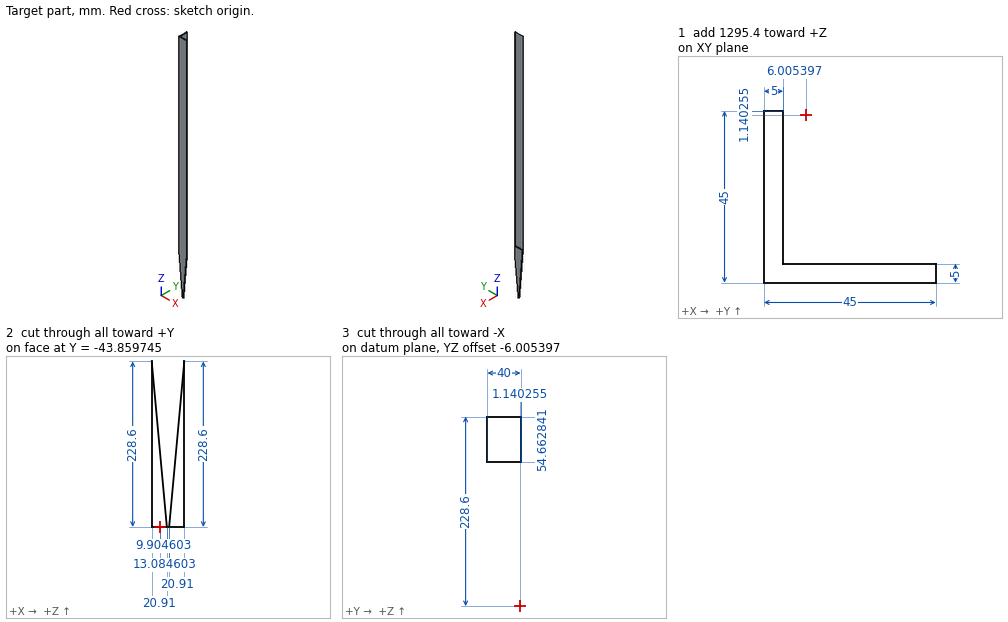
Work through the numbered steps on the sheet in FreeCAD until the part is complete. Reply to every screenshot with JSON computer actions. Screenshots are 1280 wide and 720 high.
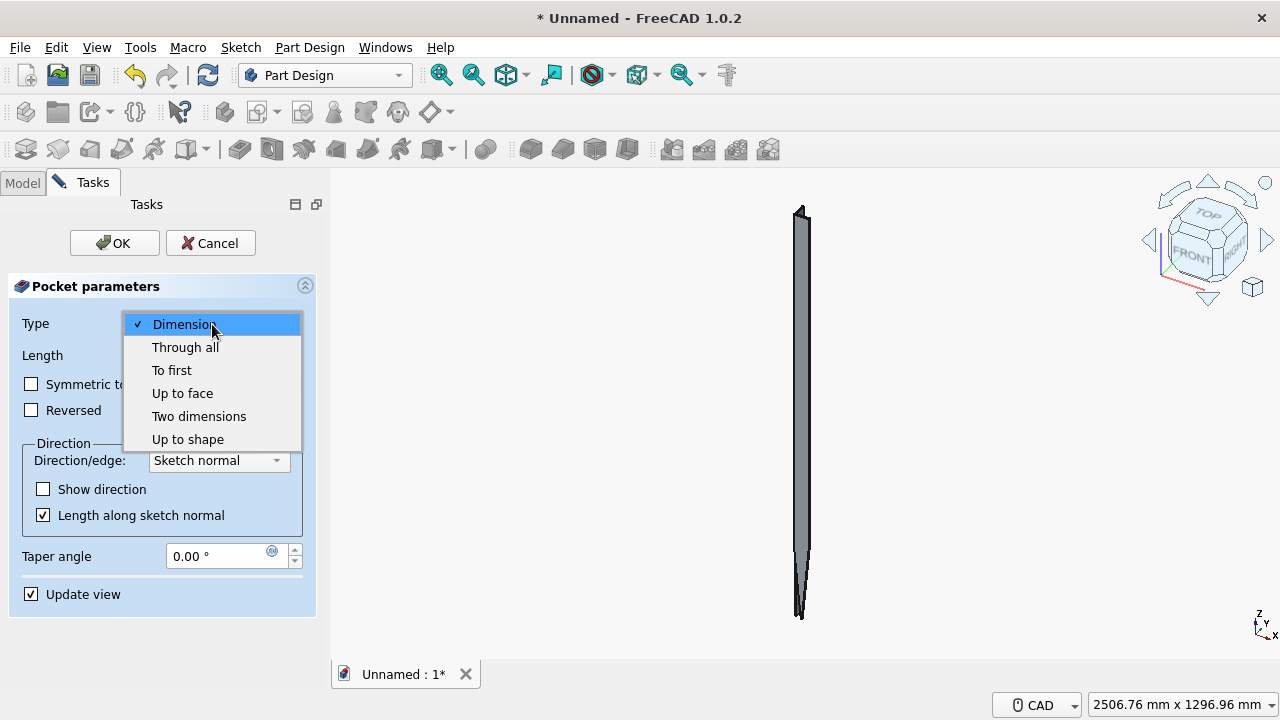
{"action": "left_click", "coordinate": [212, 348]}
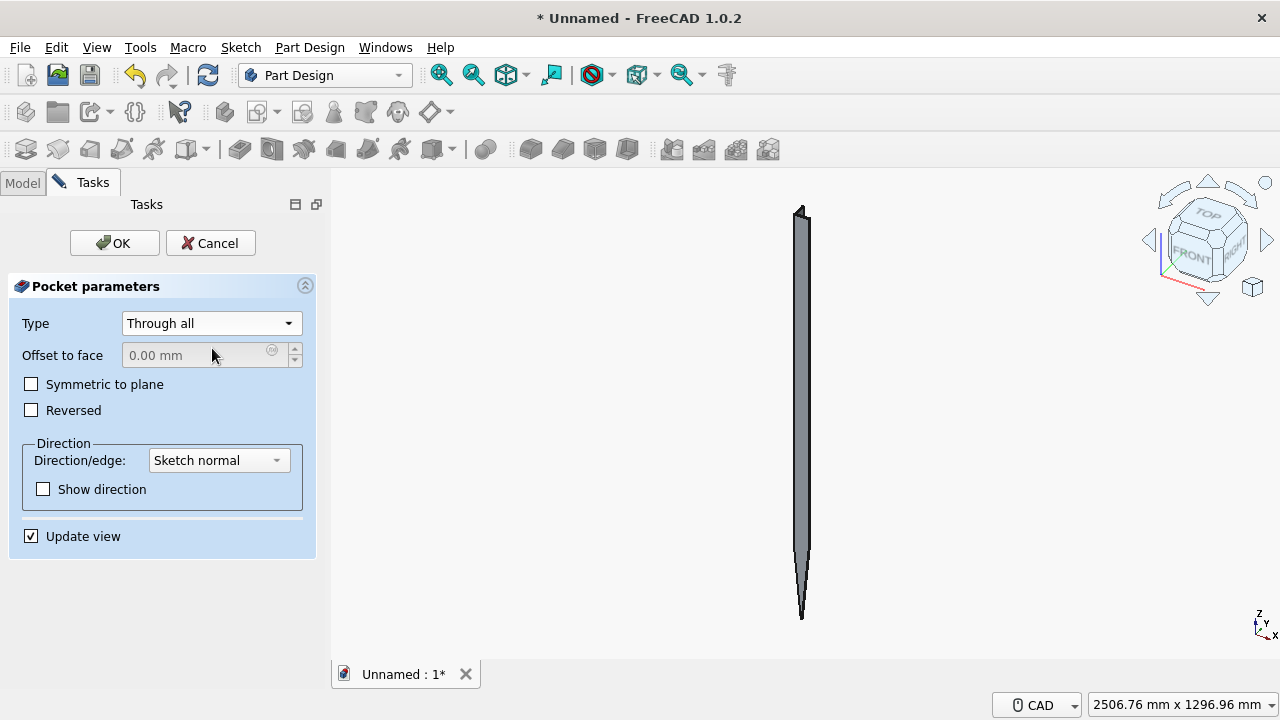
{"action": "left_click", "coordinate": [115, 243]}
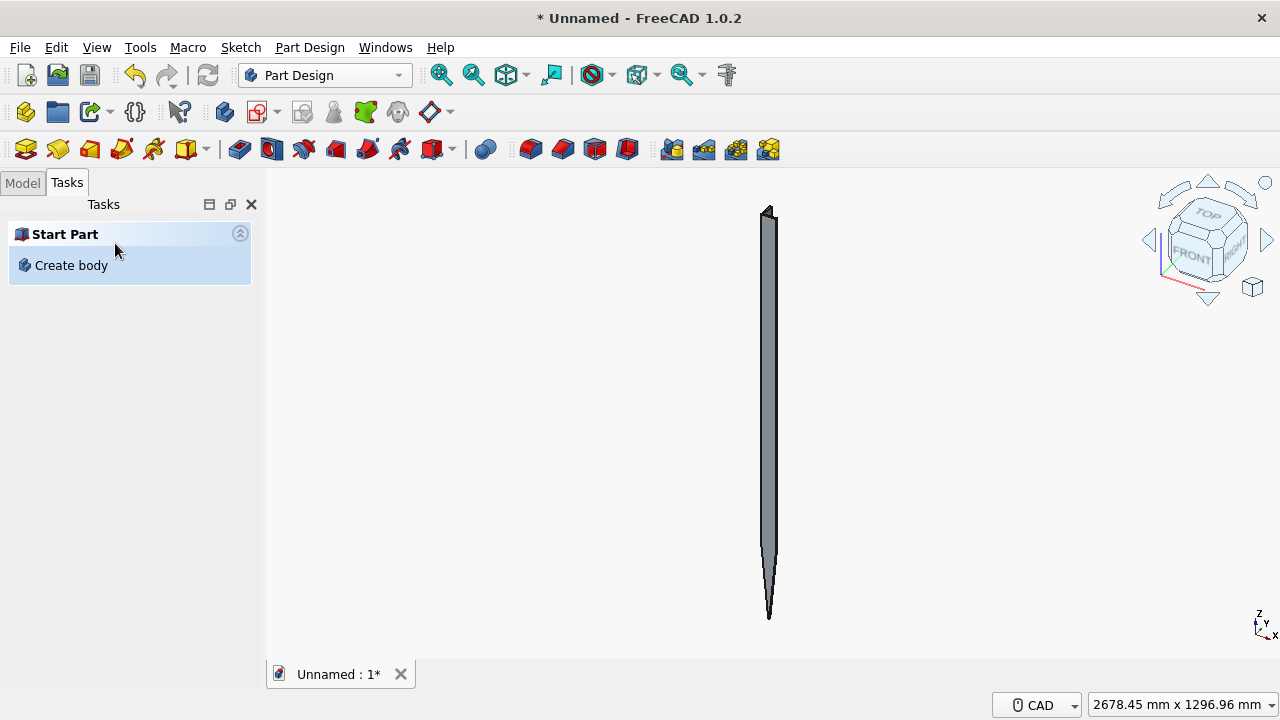
{"action": "key", "text": "0"}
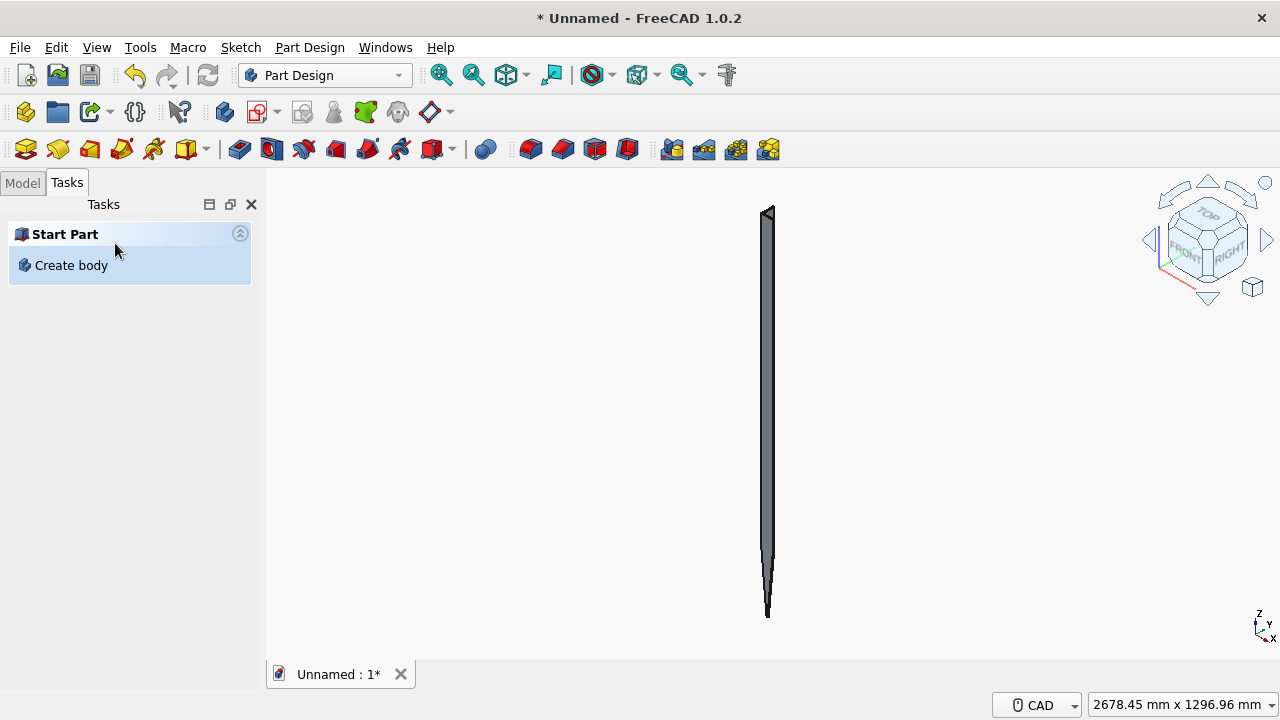
{"action": "key", "text": "3"}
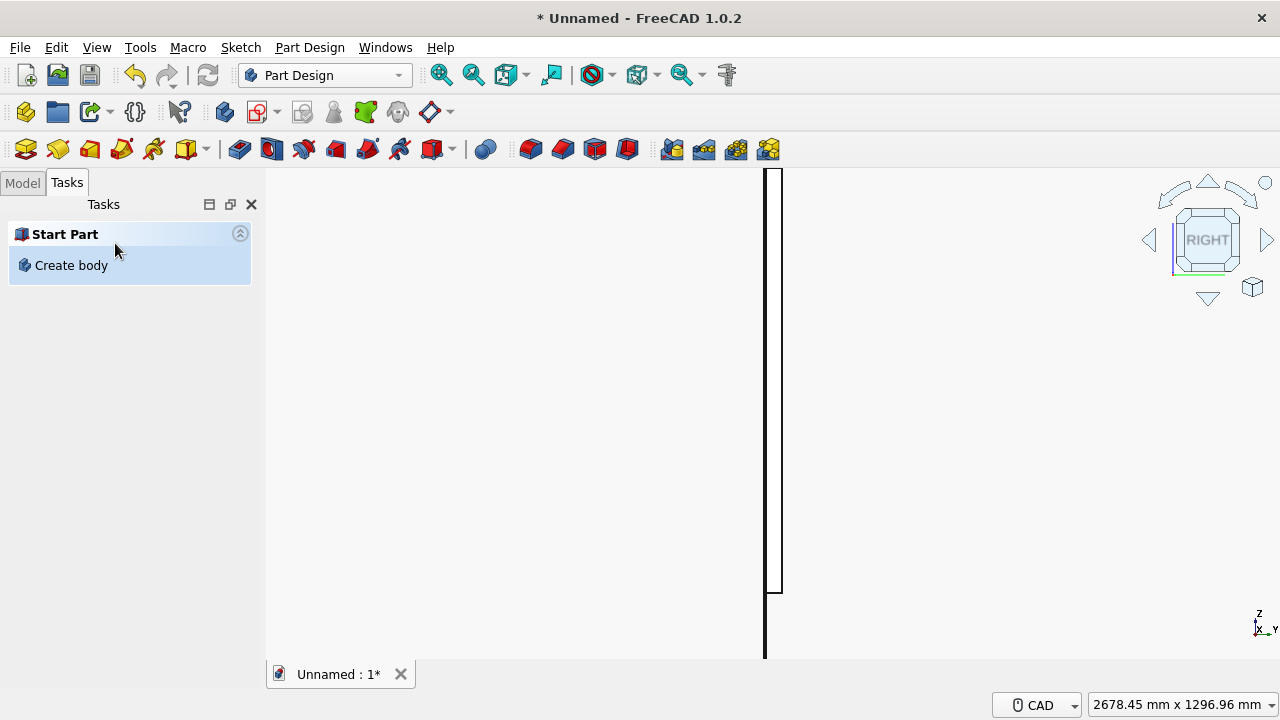
{"action": "key", "text": "v f"}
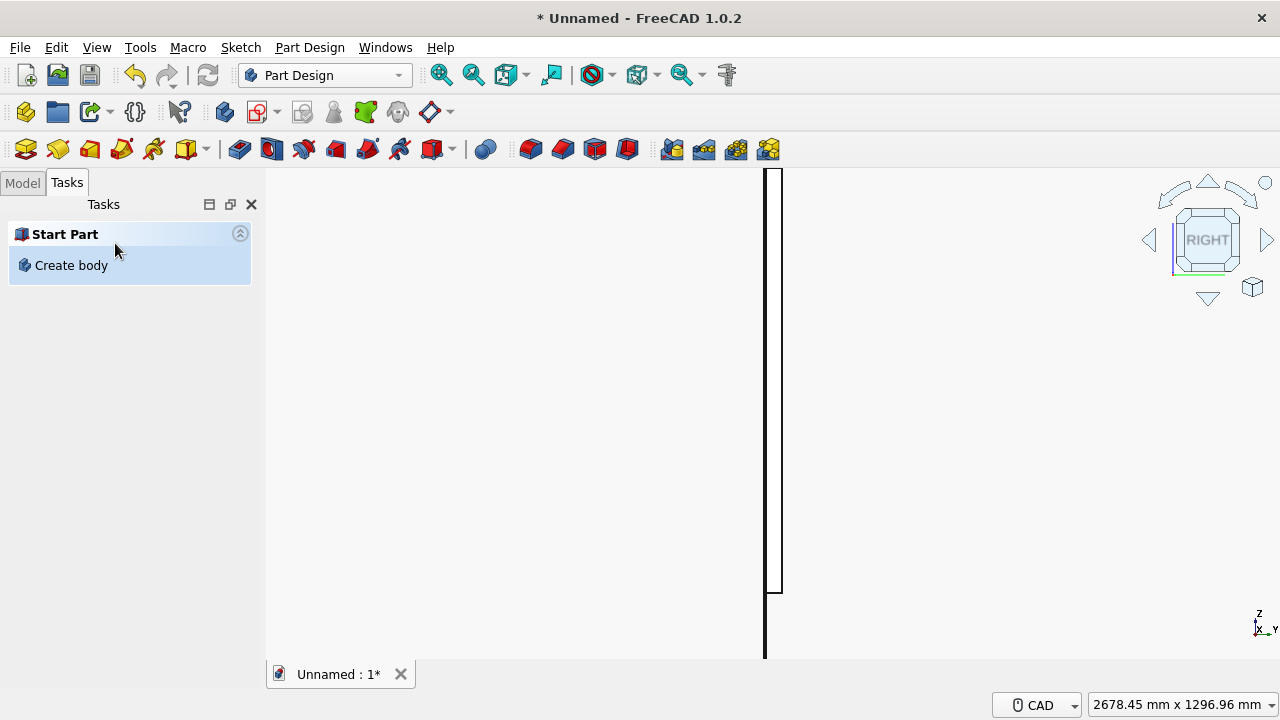
{"action": "key", "text": "2"}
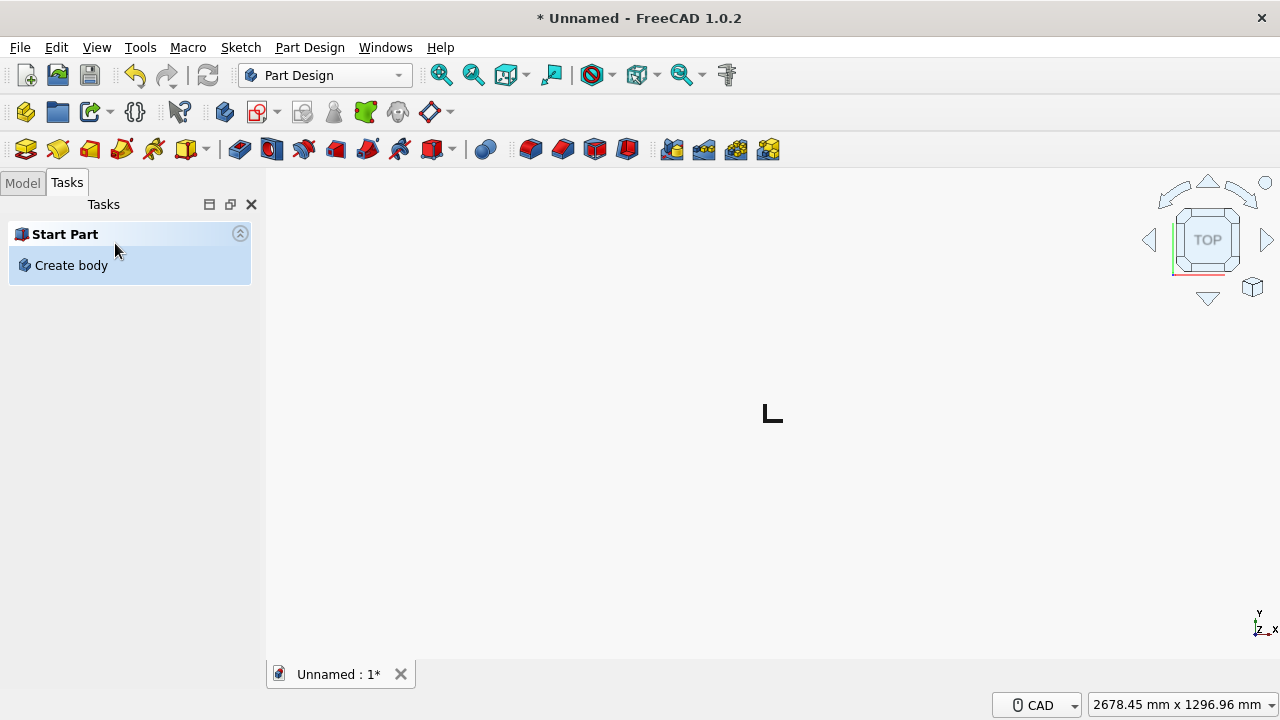
{"action": "key", "text": "v f"}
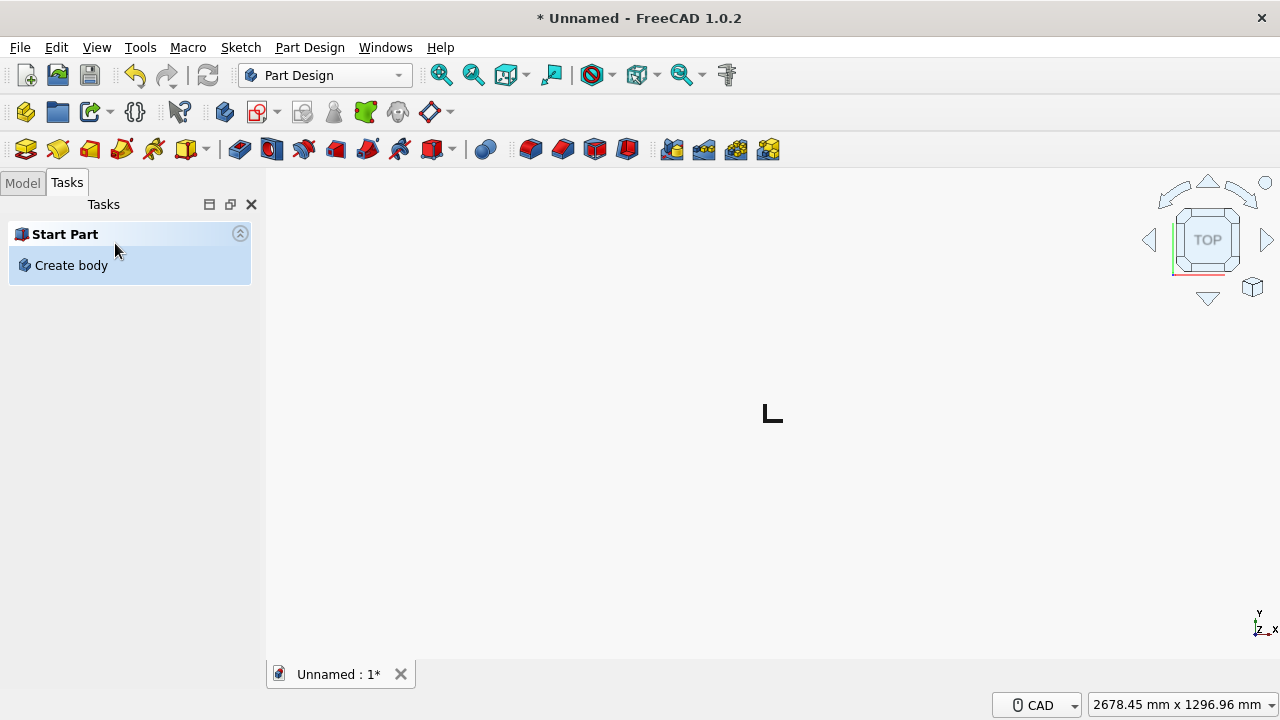
{"action": "left_click", "coordinate": [23, 182]}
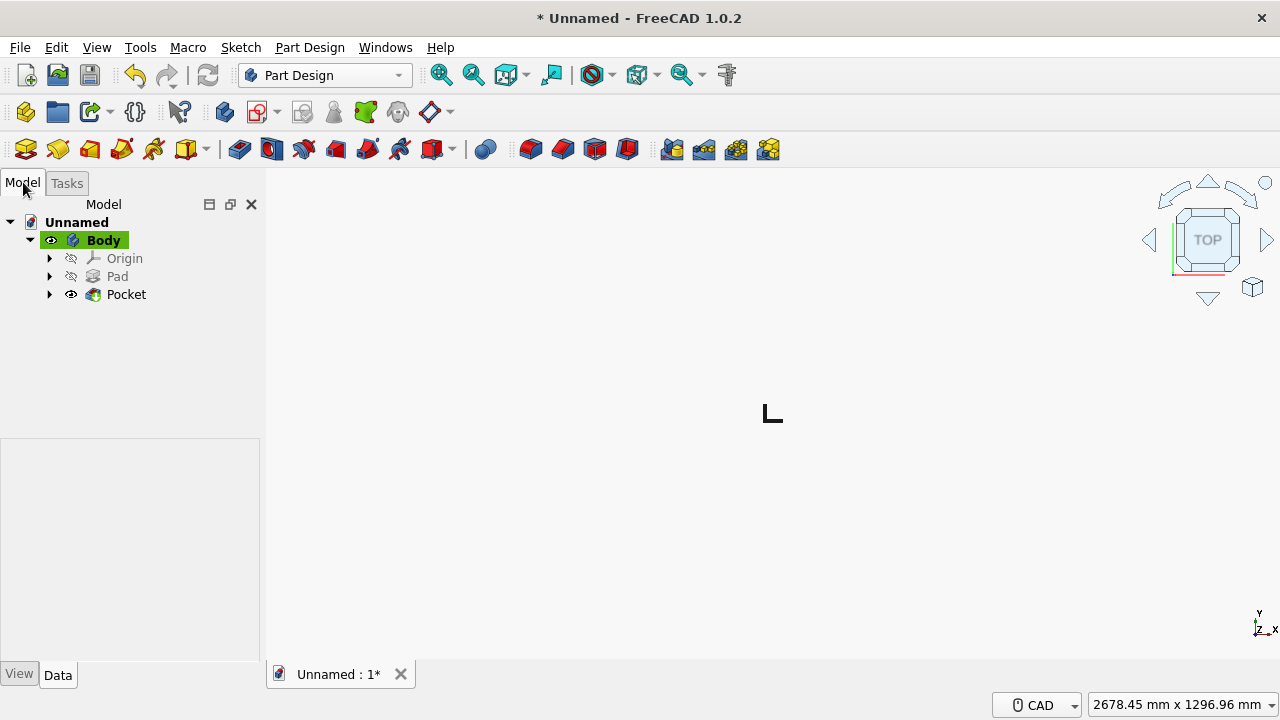
{"action": "left_click", "coordinate": [50, 258]}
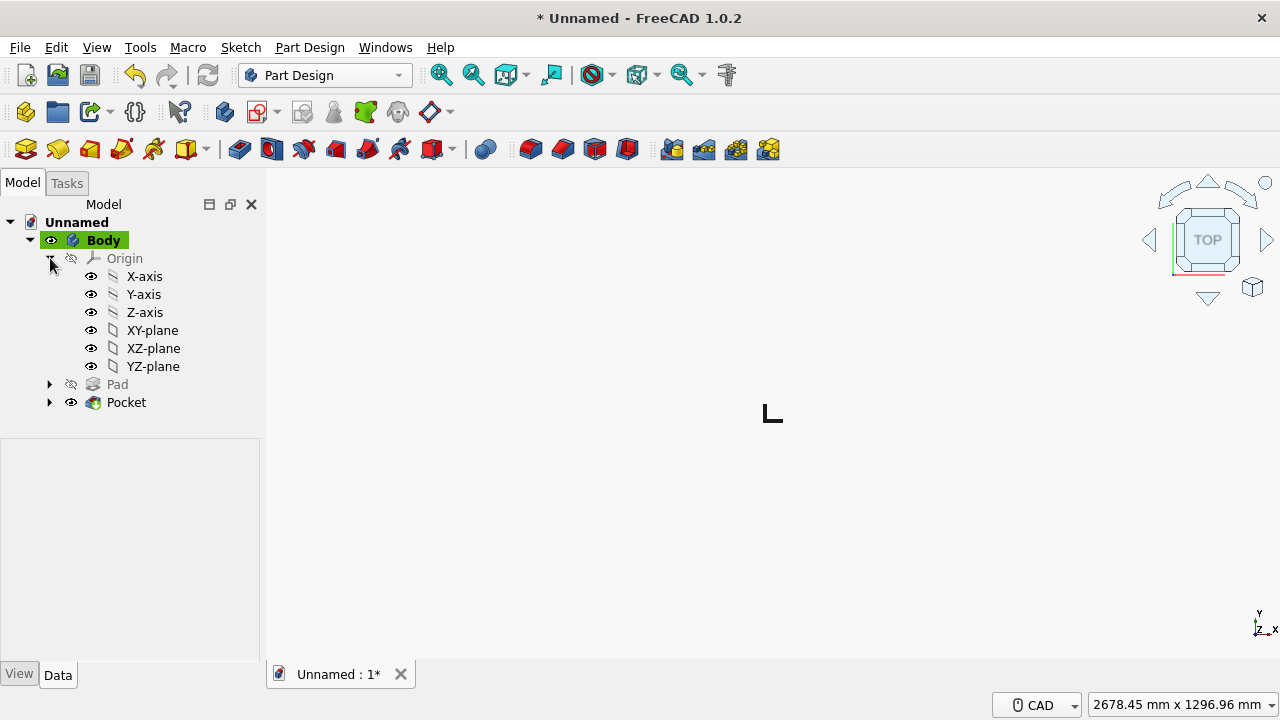
{"action": "left_click", "coordinate": [136, 366]}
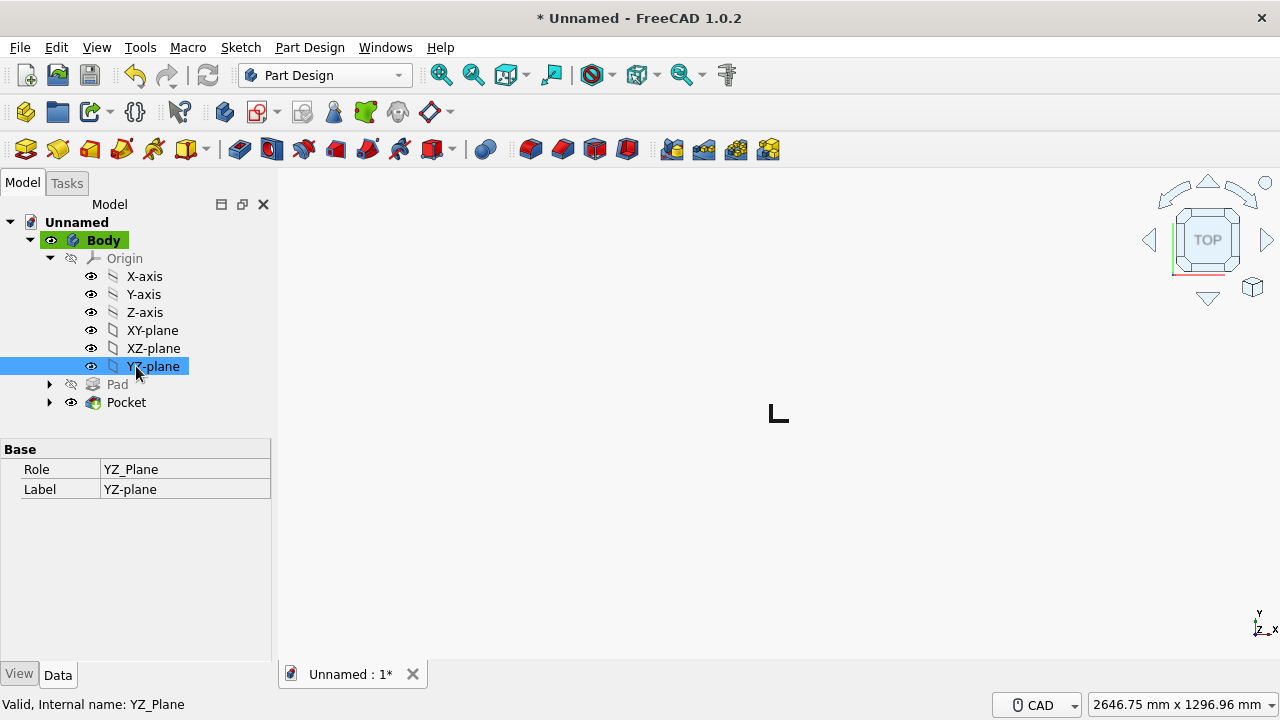
{"action": "left_click", "coordinate": [430, 112]}